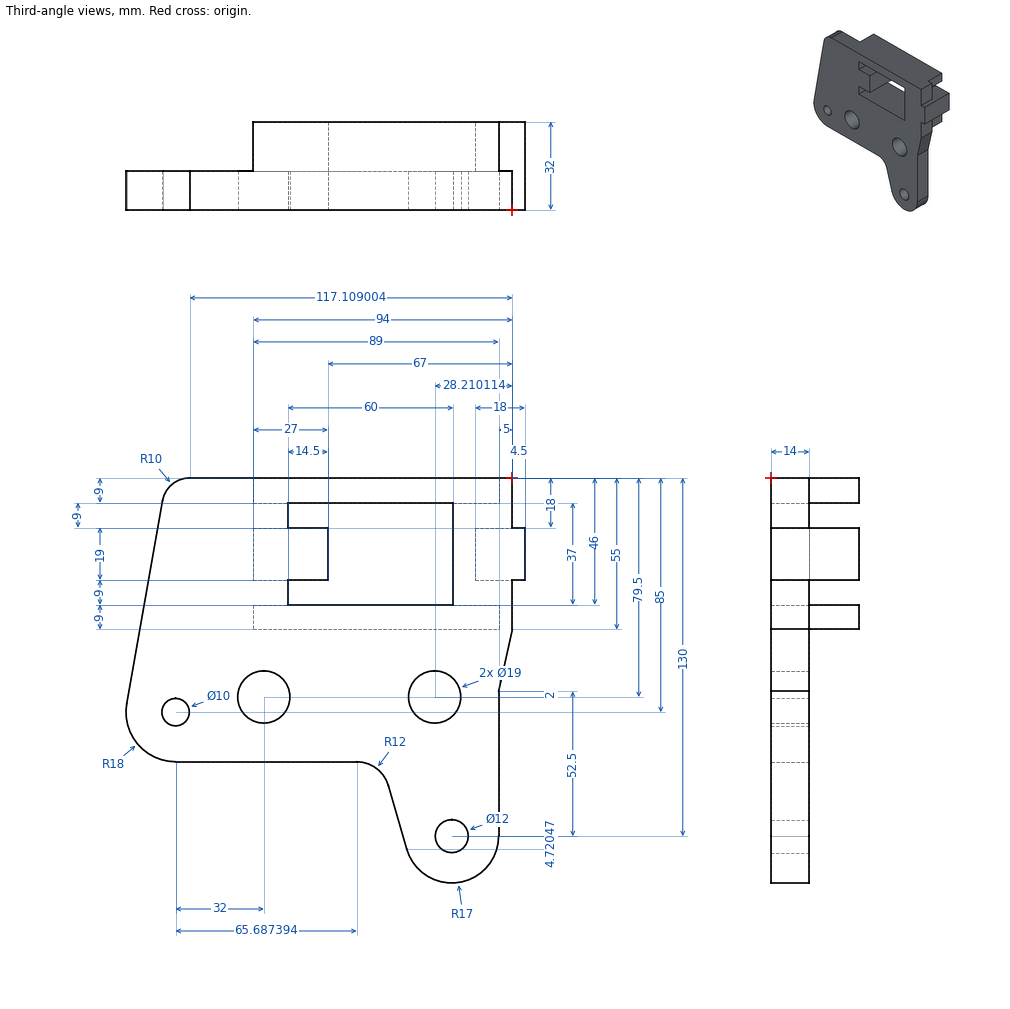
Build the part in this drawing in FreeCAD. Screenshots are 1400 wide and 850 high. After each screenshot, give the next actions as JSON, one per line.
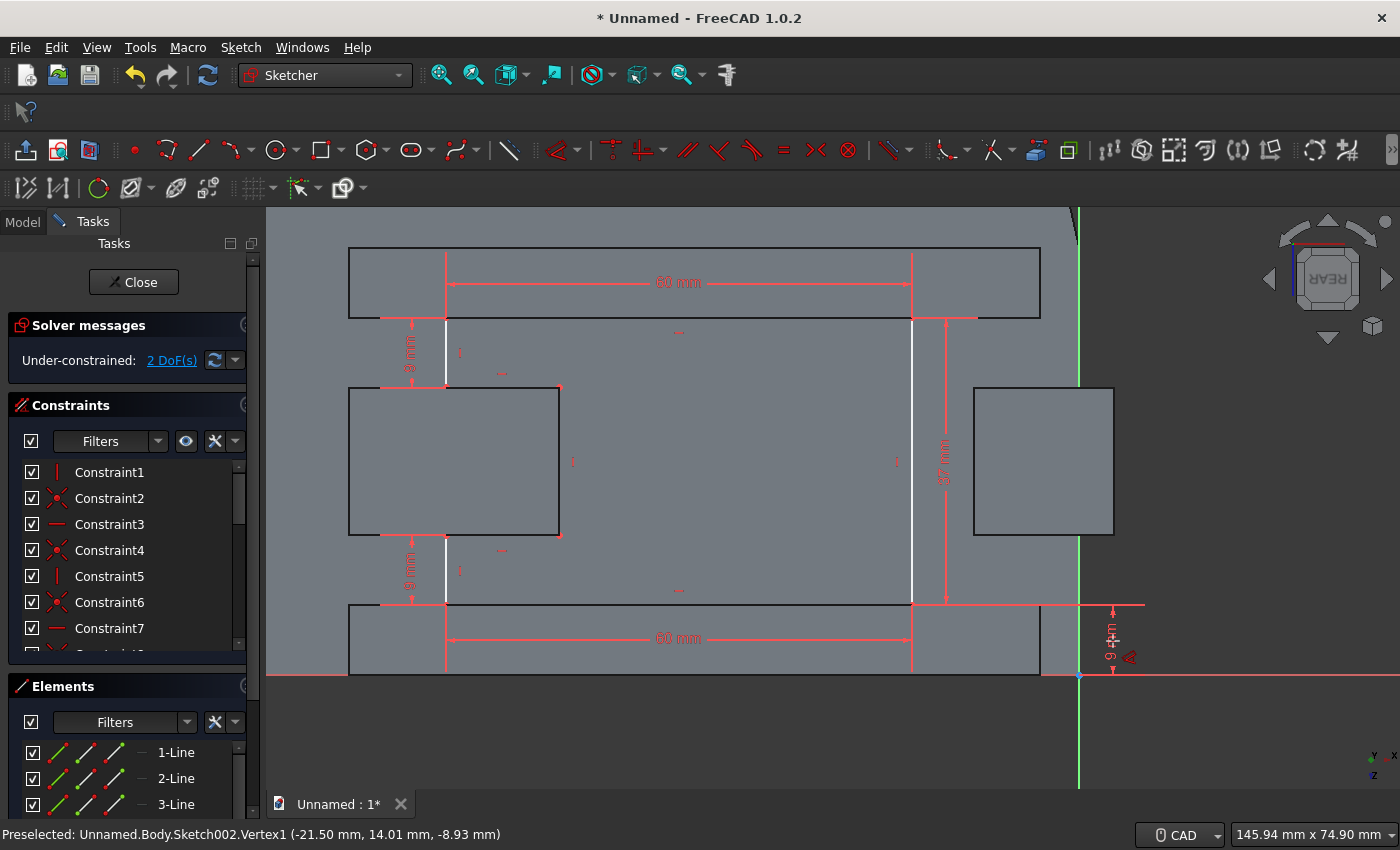
{"action": "left_click", "coordinate": [559, 388]}
{"action": "left_click", "coordinate": [819, 709]}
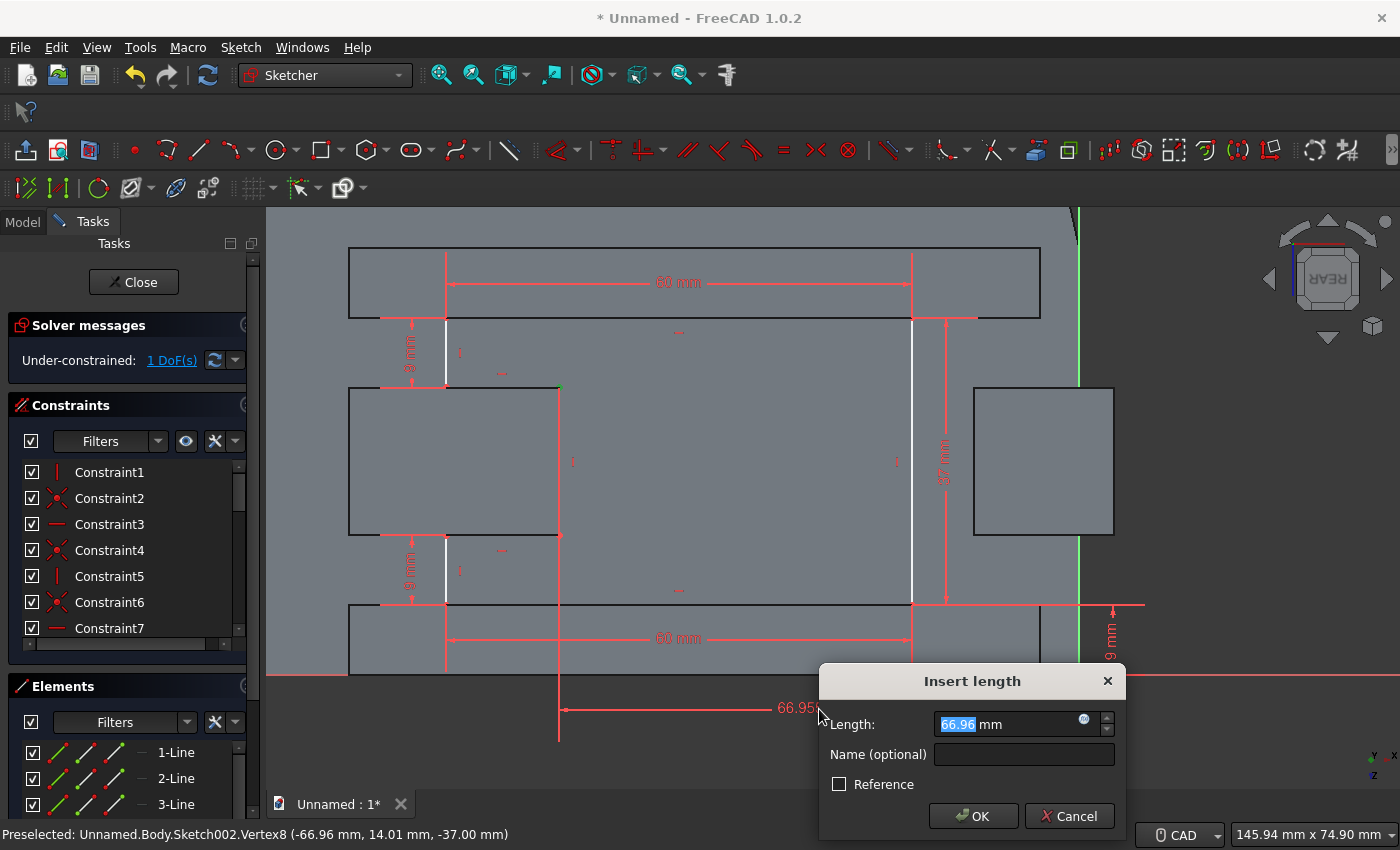
{"action": "type", "text": "67"}
{"action": "key", "text": "Return"}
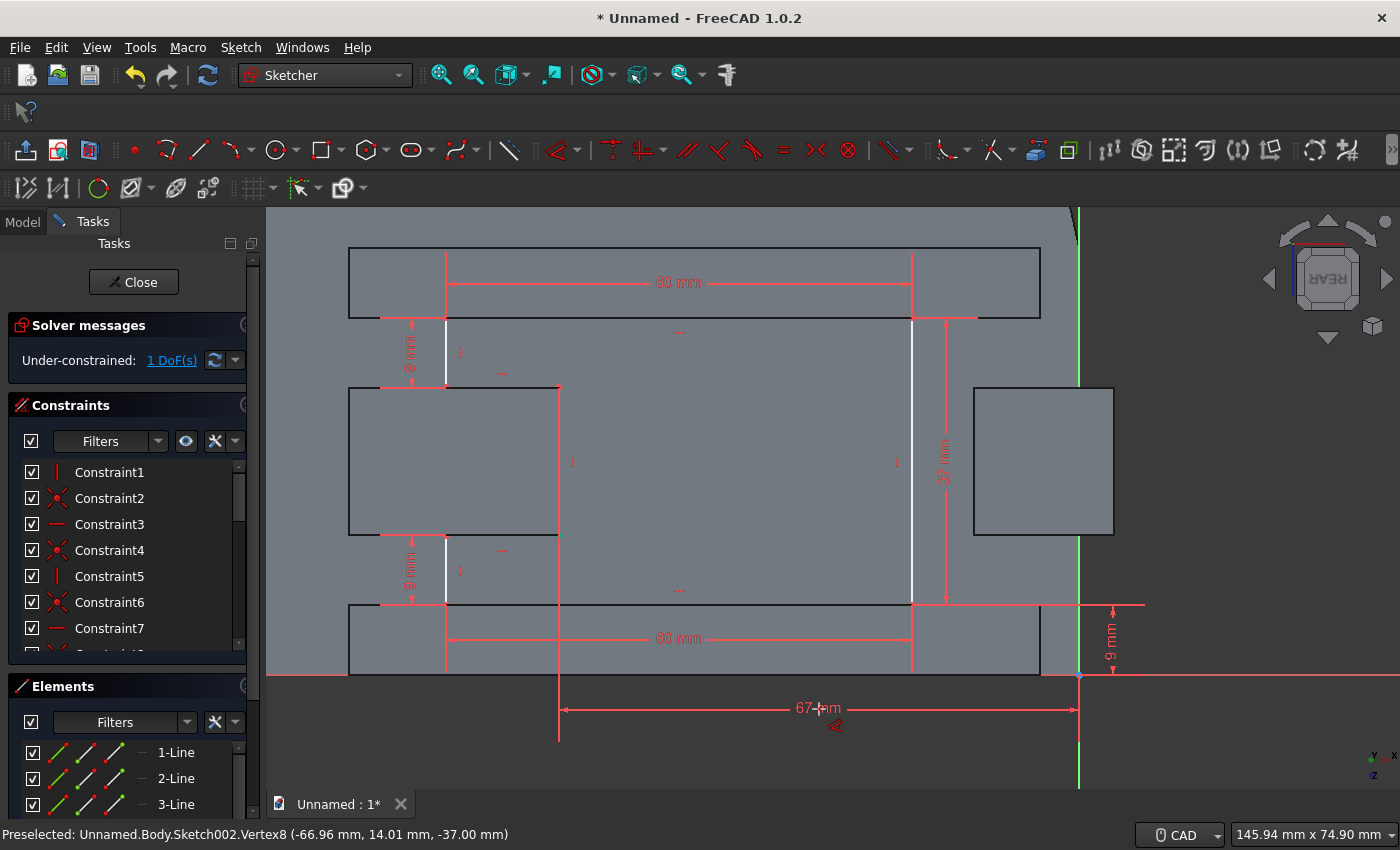
{"action": "left_click", "coordinate": [480, 388]}
{"action": "left_click", "coordinate": [502, 354]}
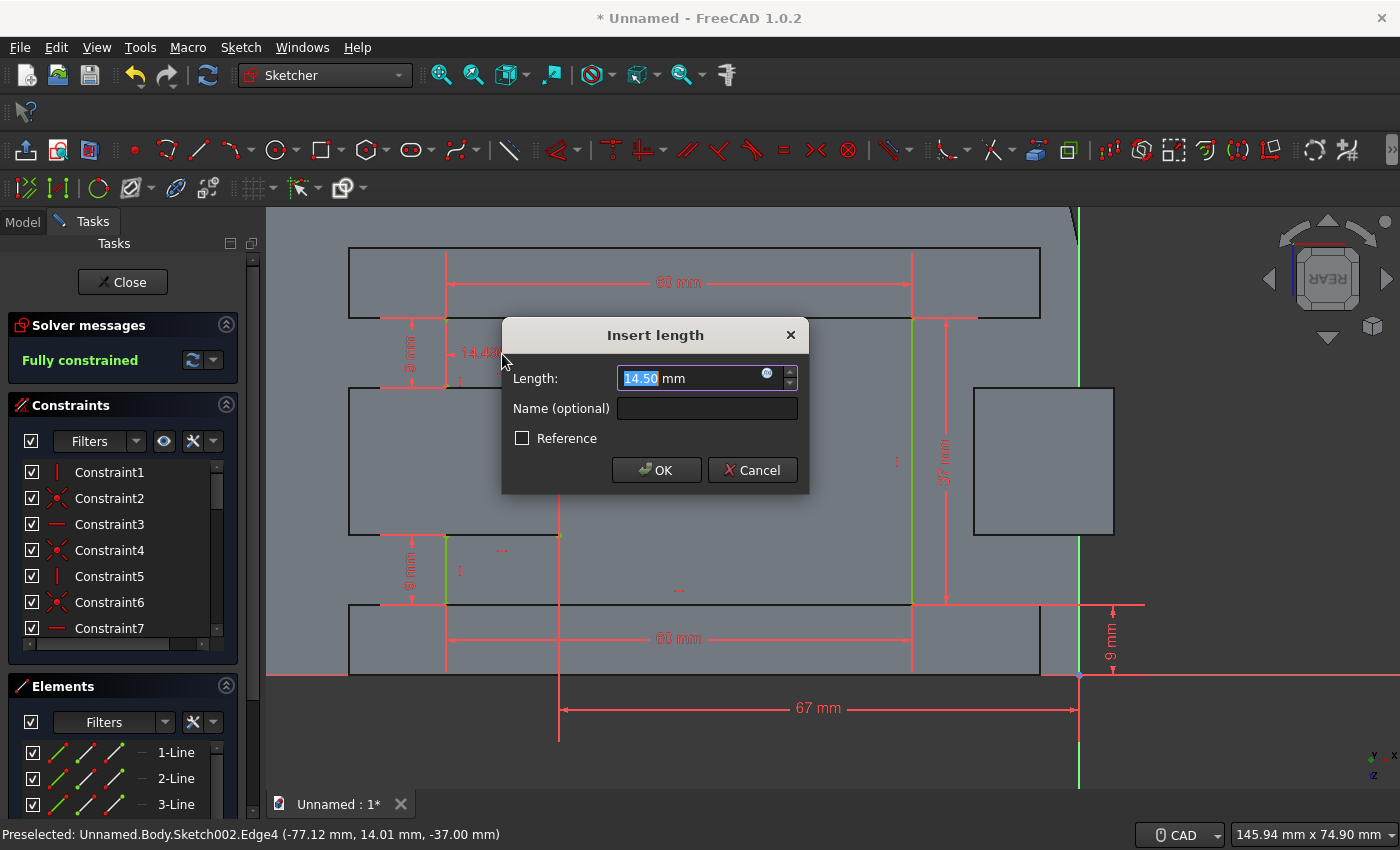
{"action": "type", "text": "14.5"}
{"action": "key", "text": "Return"}
{"action": "key", "text": "Escape"}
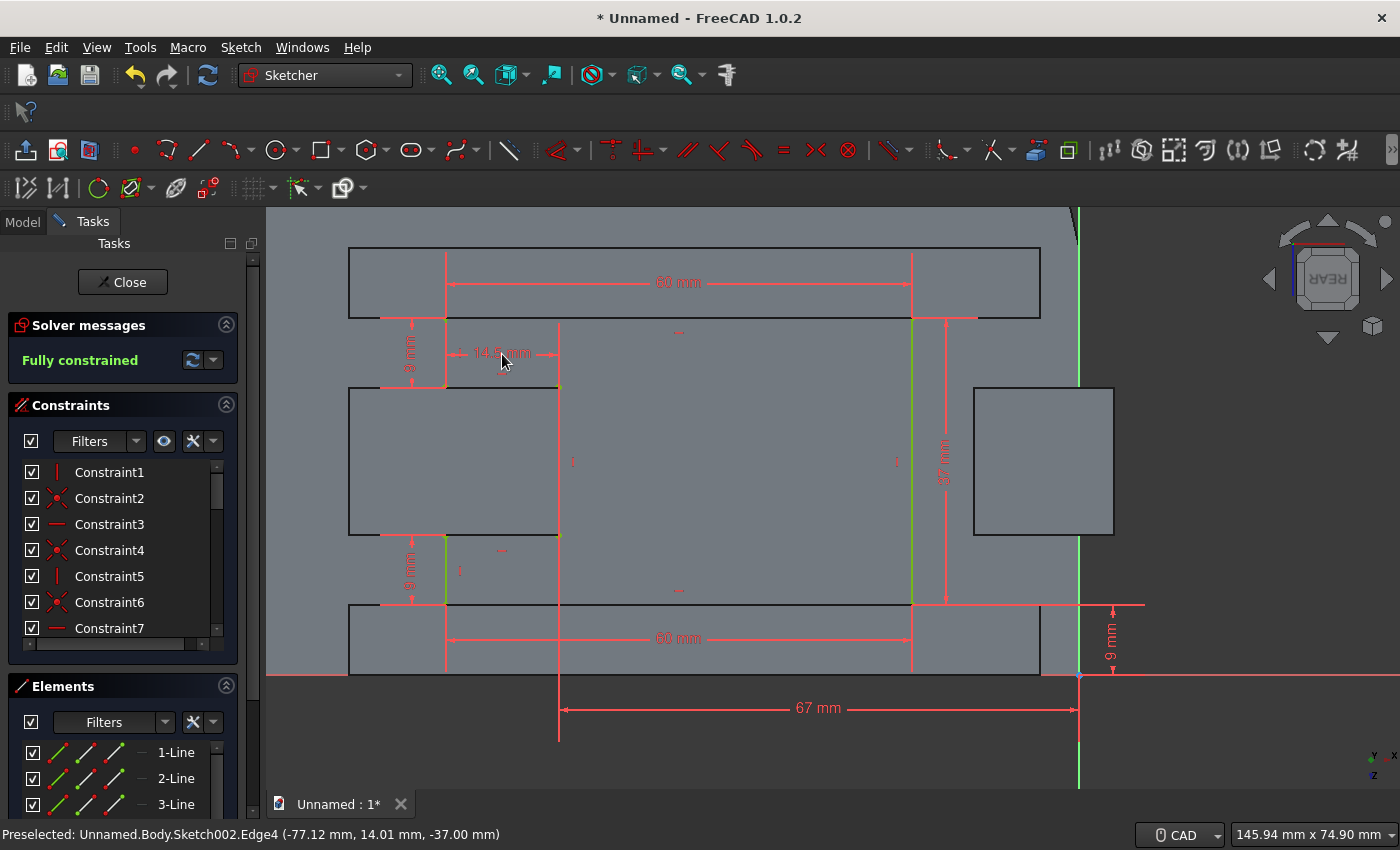
{"action": "left_click", "coordinate": [123, 282]}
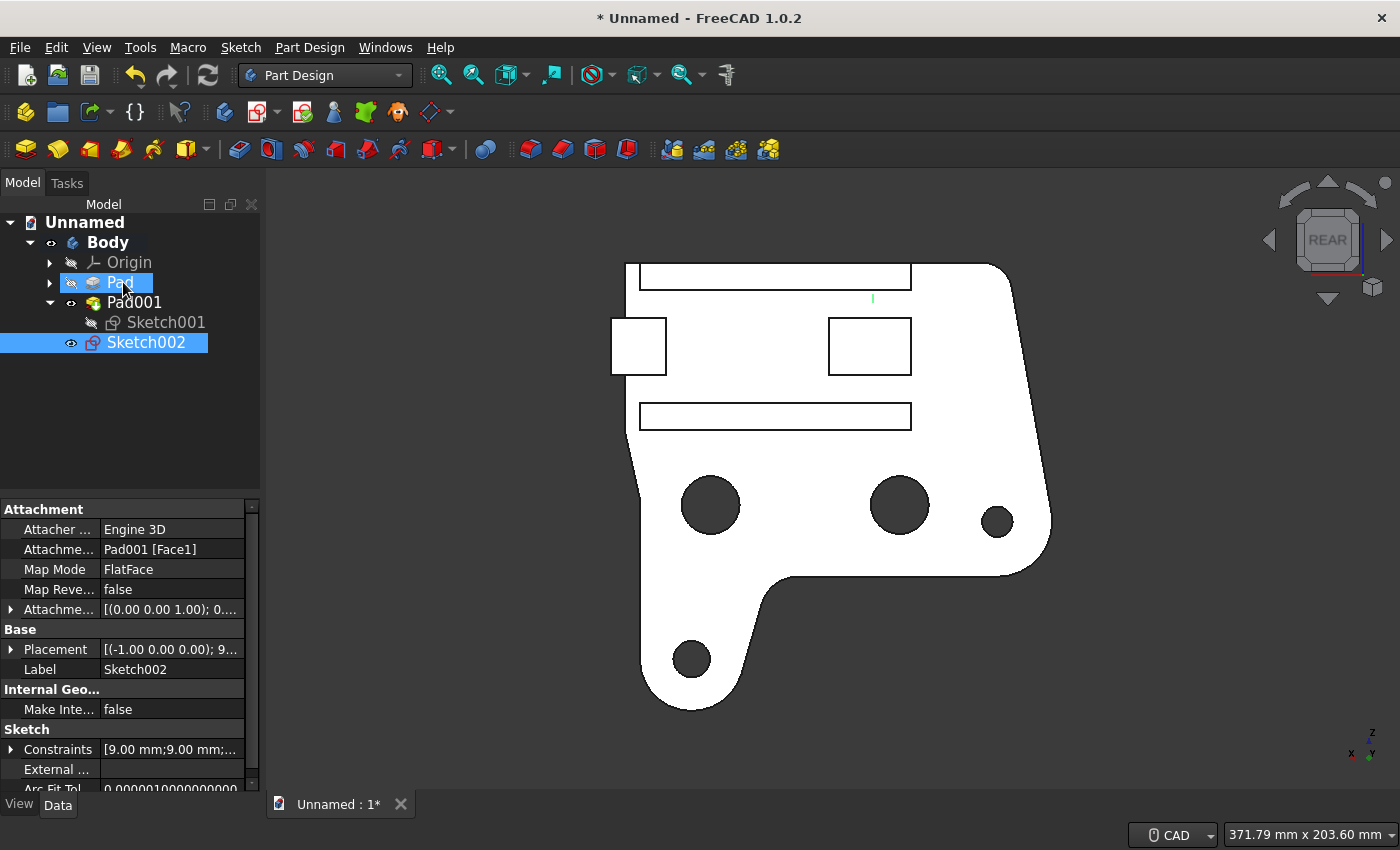
{"action": "left_click", "coordinate": [240, 150]}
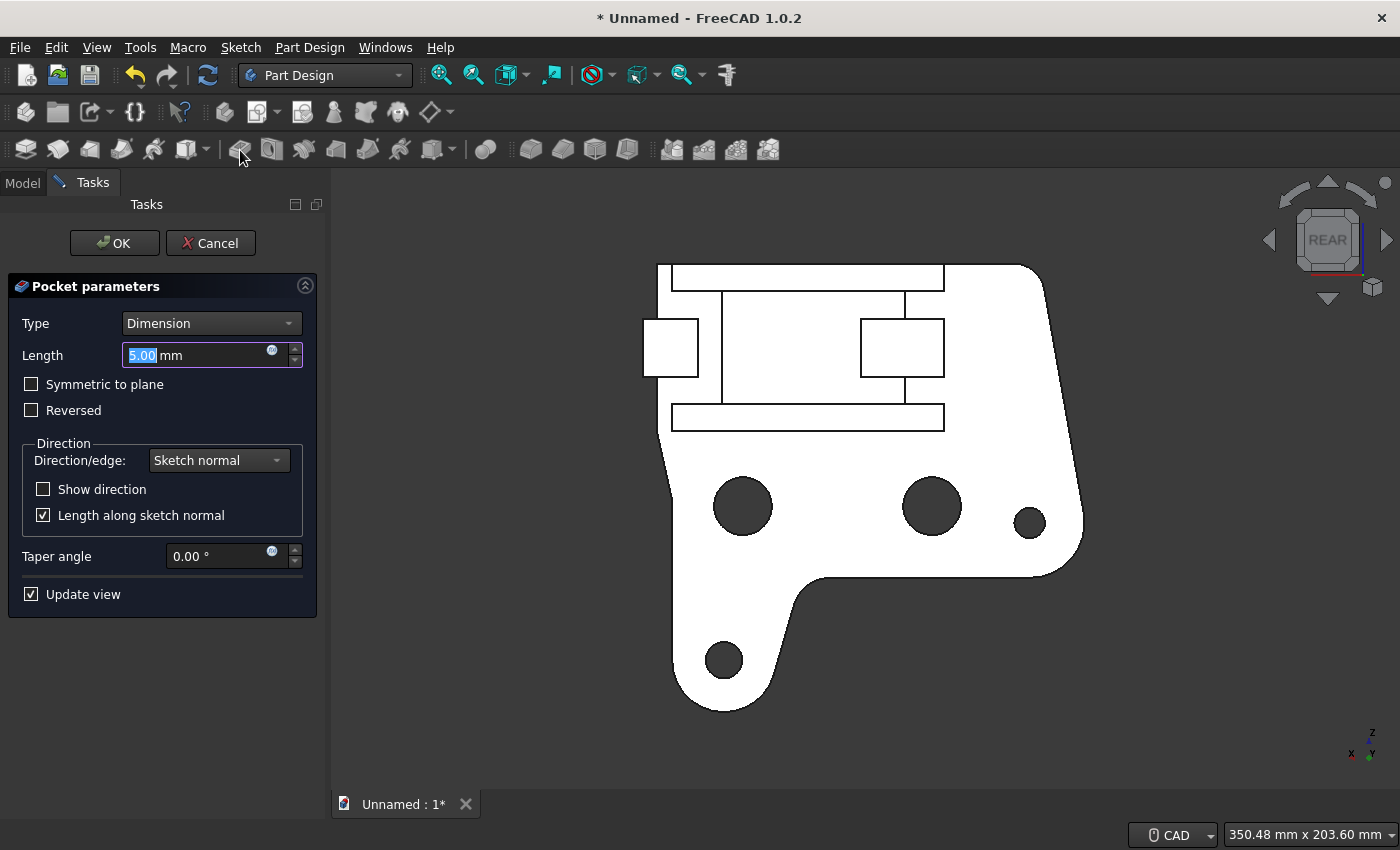
{"action": "left_click", "coordinate": [212, 324]}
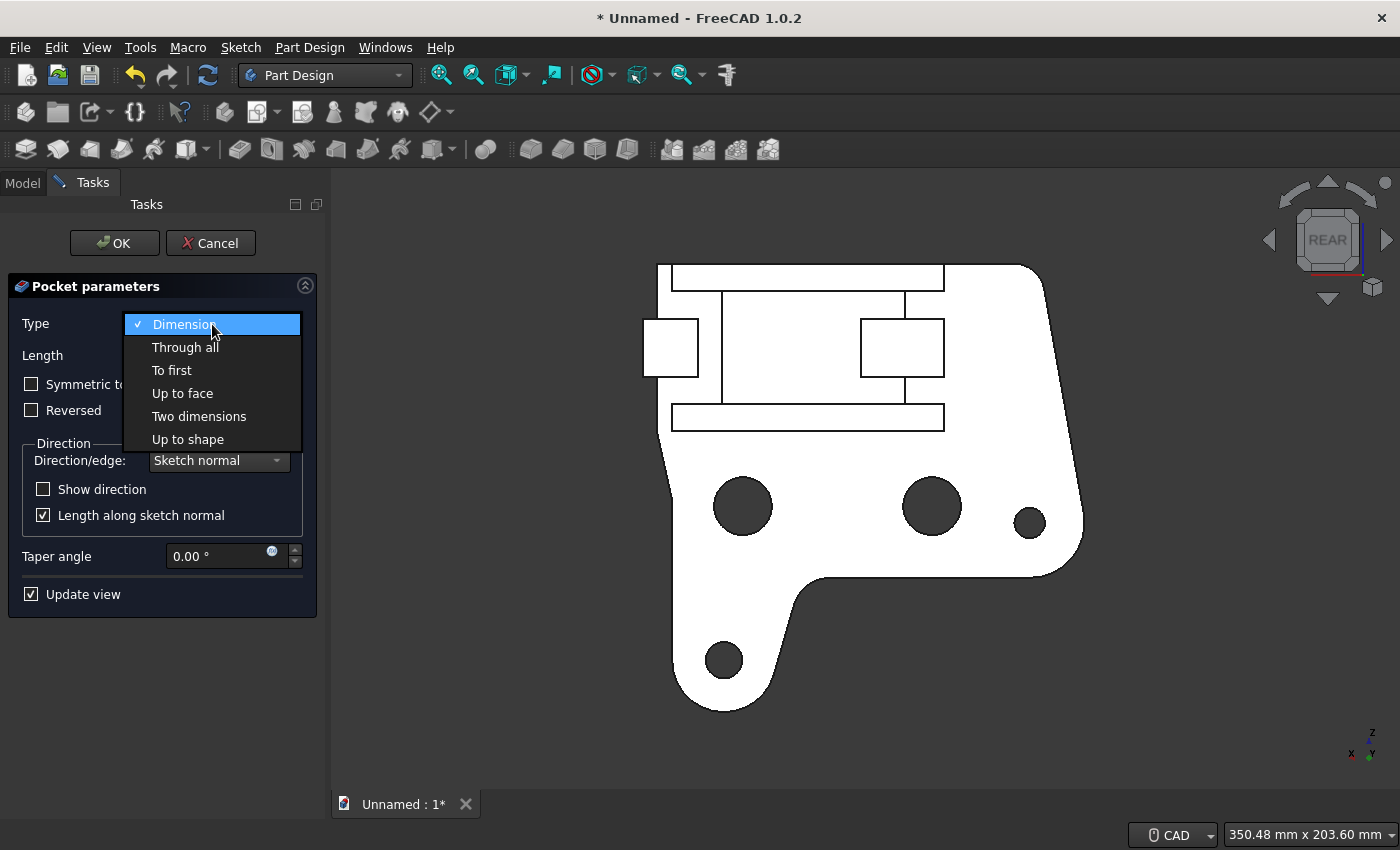
{"action": "left_click", "coordinate": [212, 370]}